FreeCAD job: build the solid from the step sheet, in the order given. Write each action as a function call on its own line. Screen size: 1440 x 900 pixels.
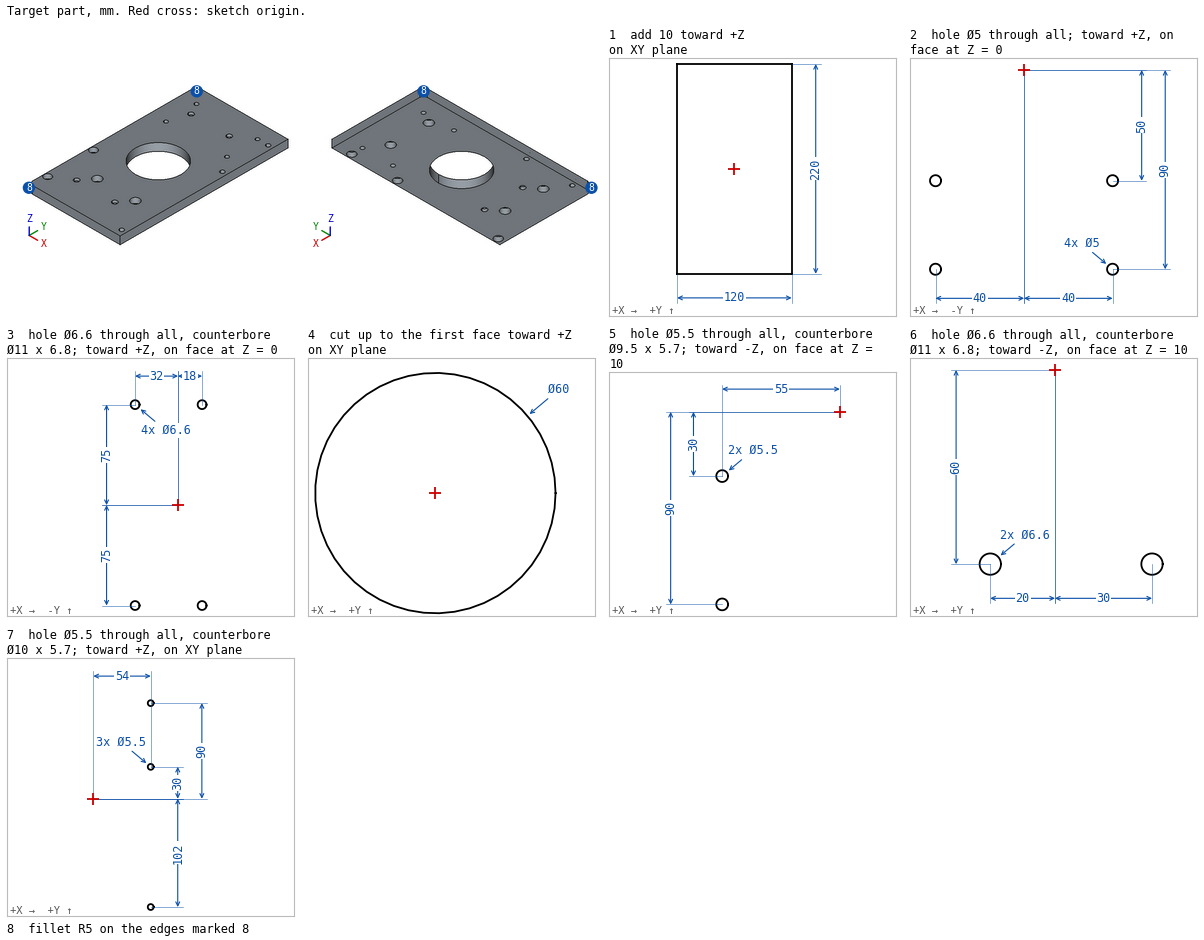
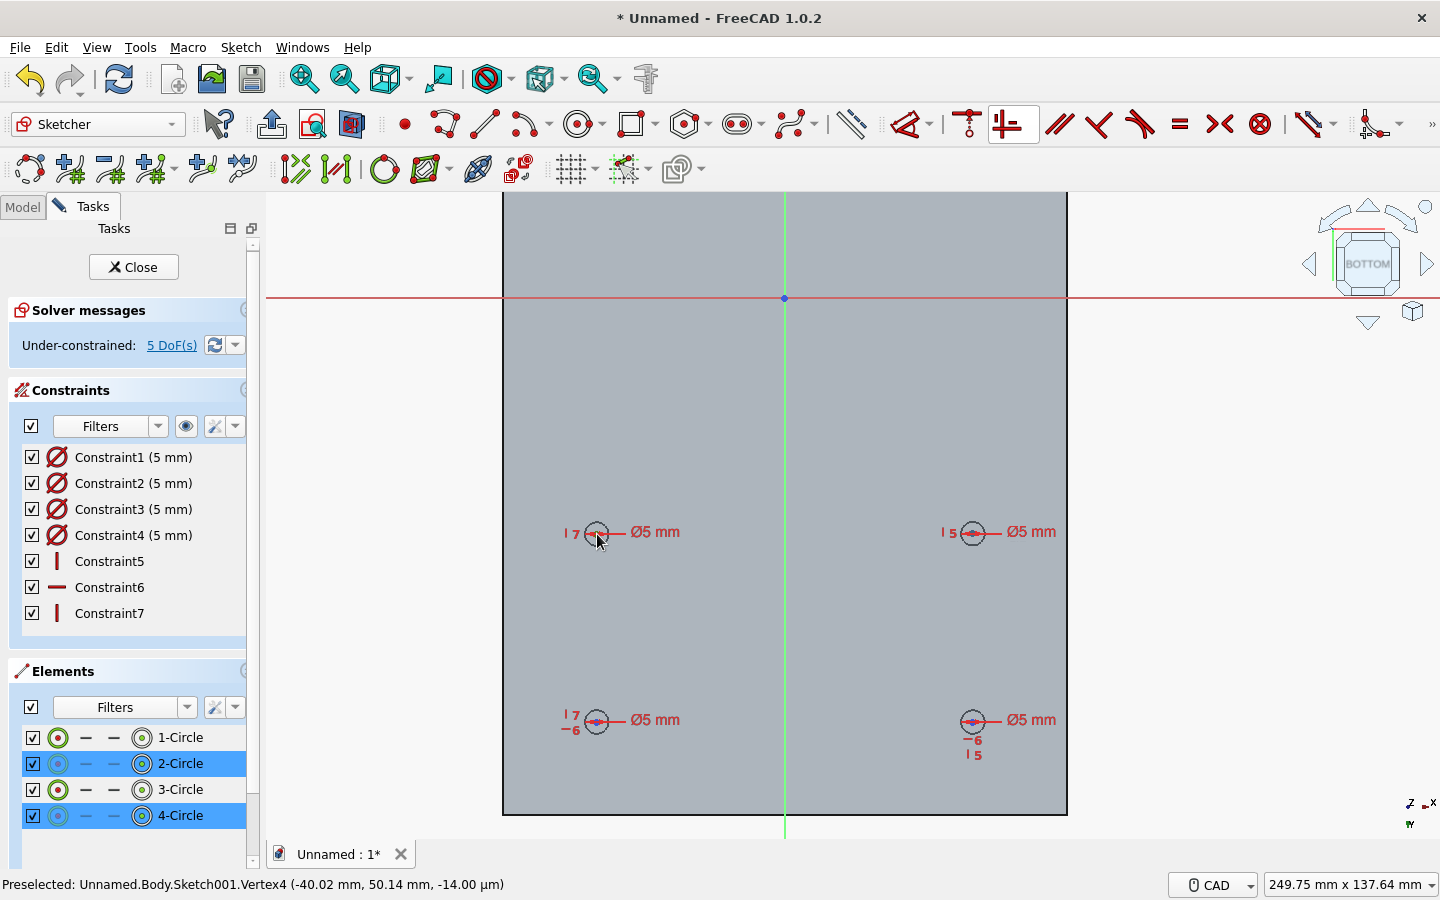
key(h)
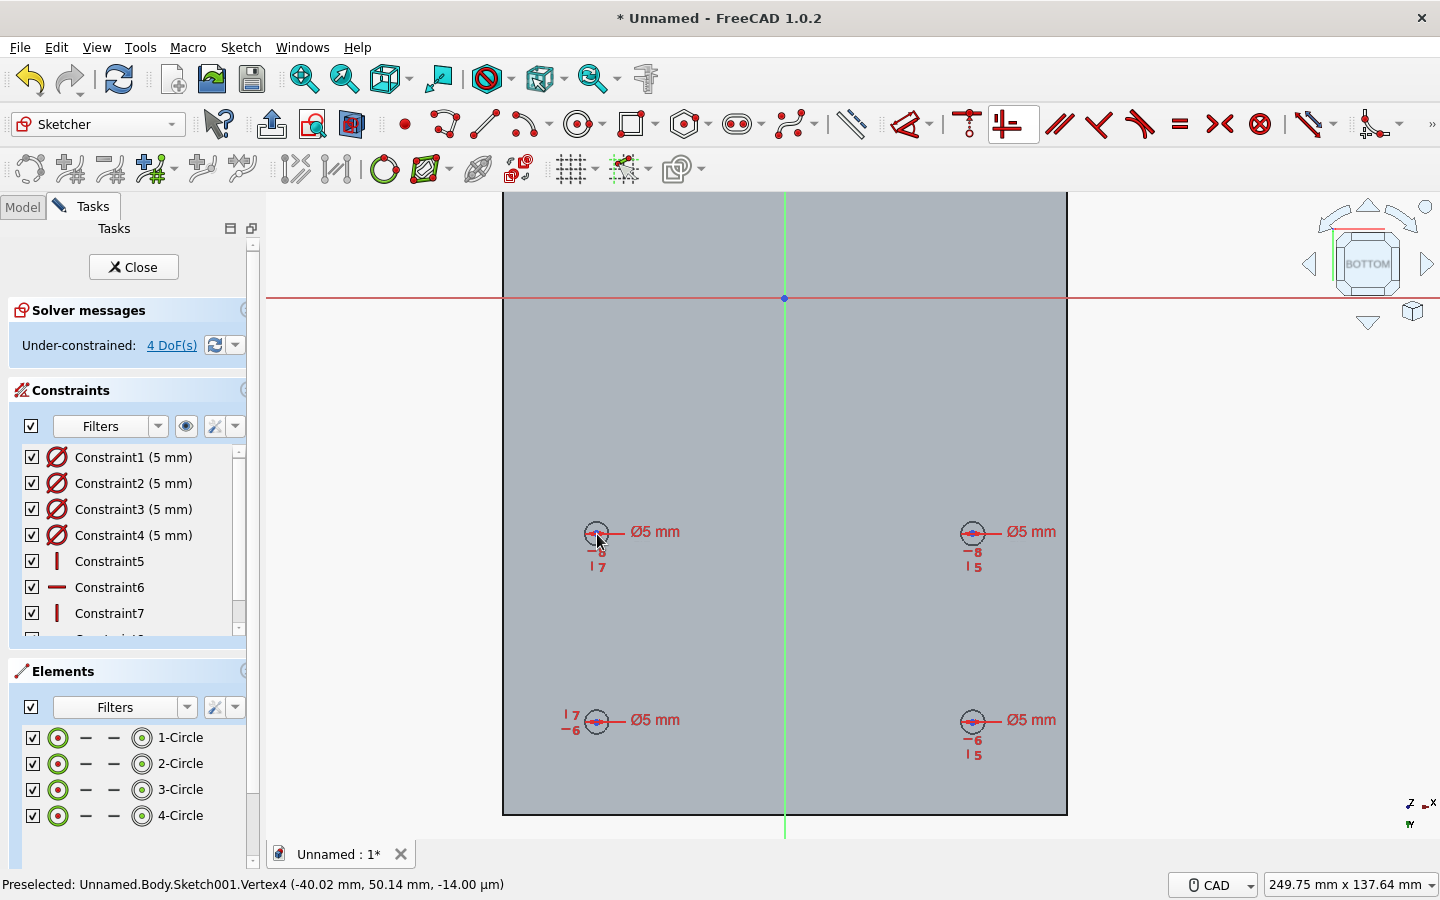
key(d)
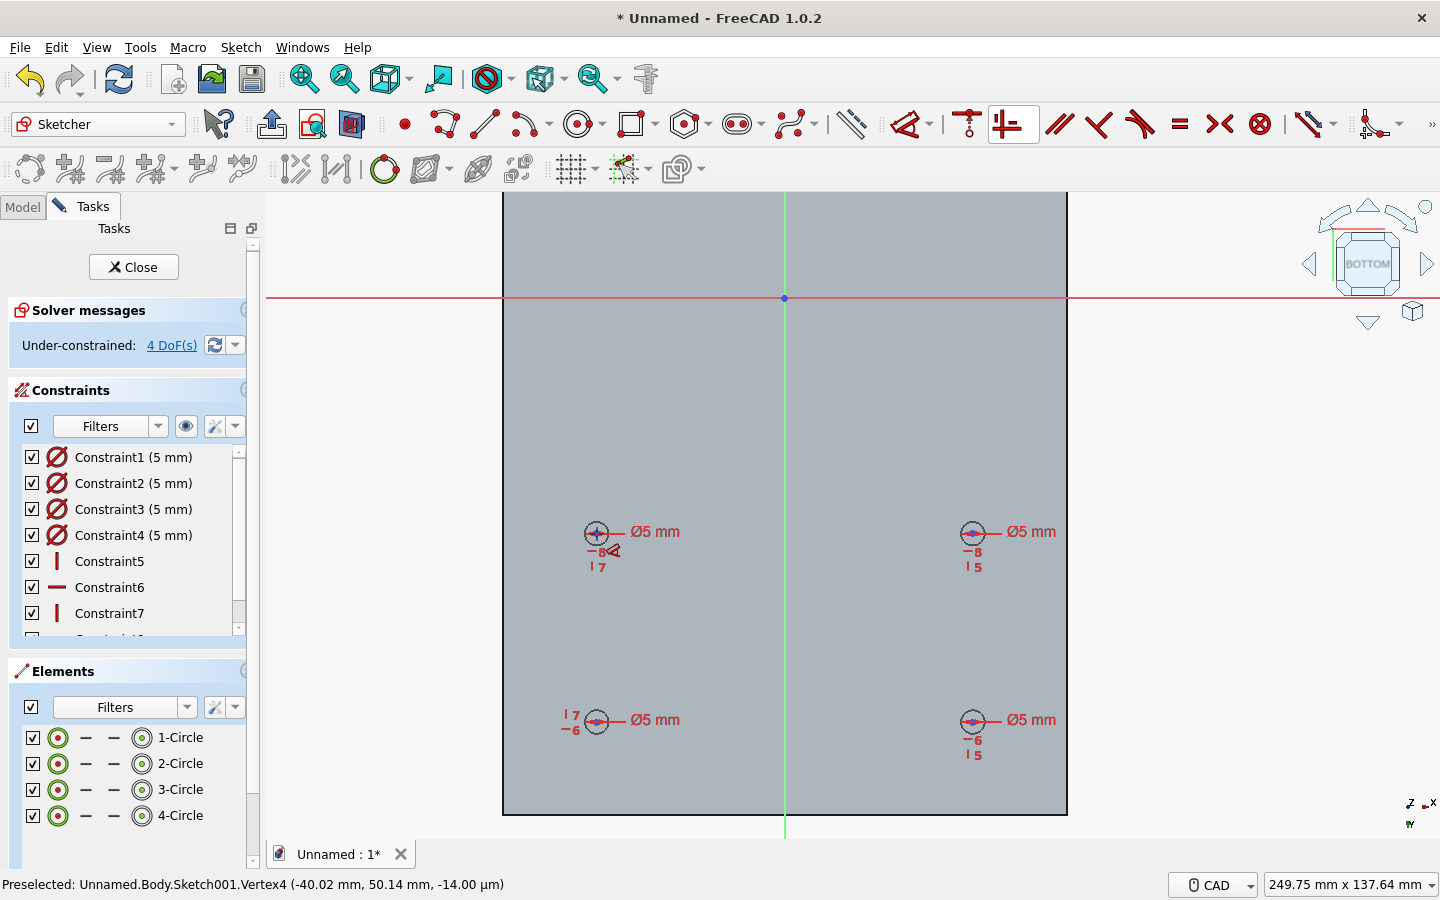
click(973, 722)
click(879, 264)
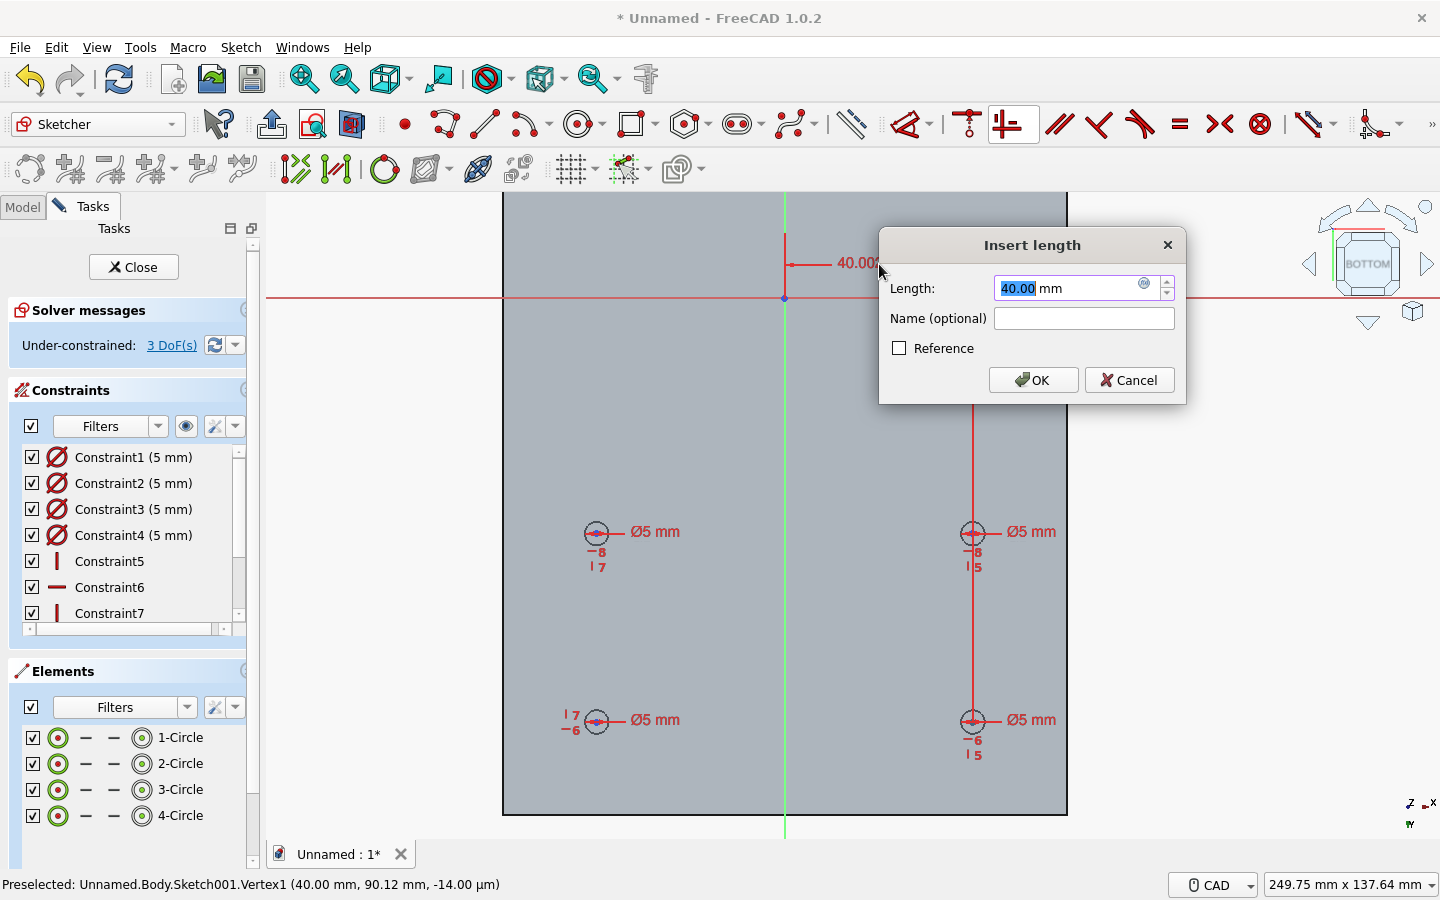
text(40)
key(Return)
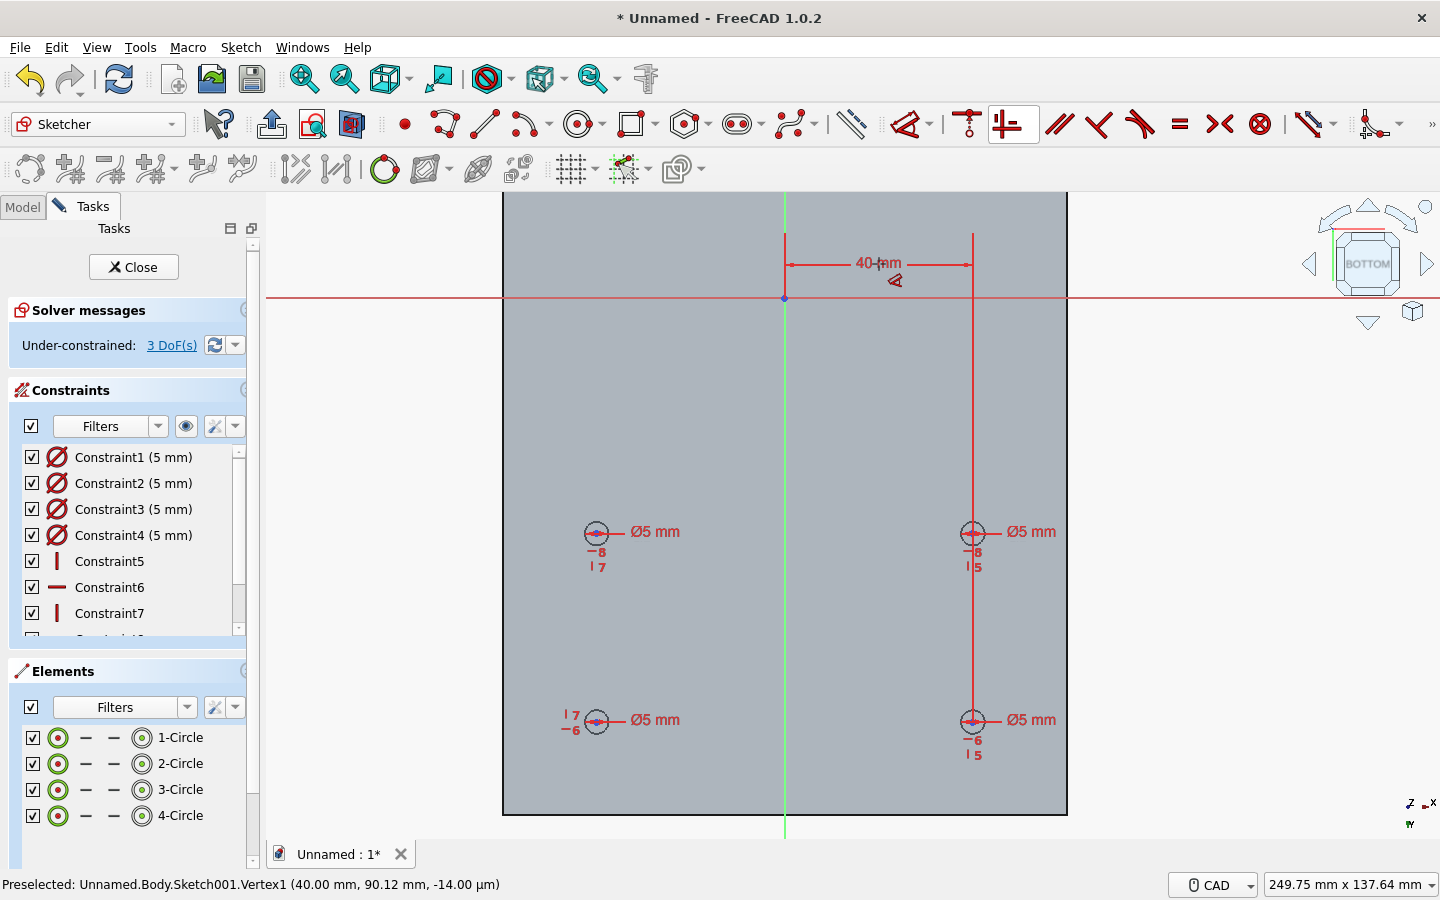
click(973, 722)
click(1007, 510)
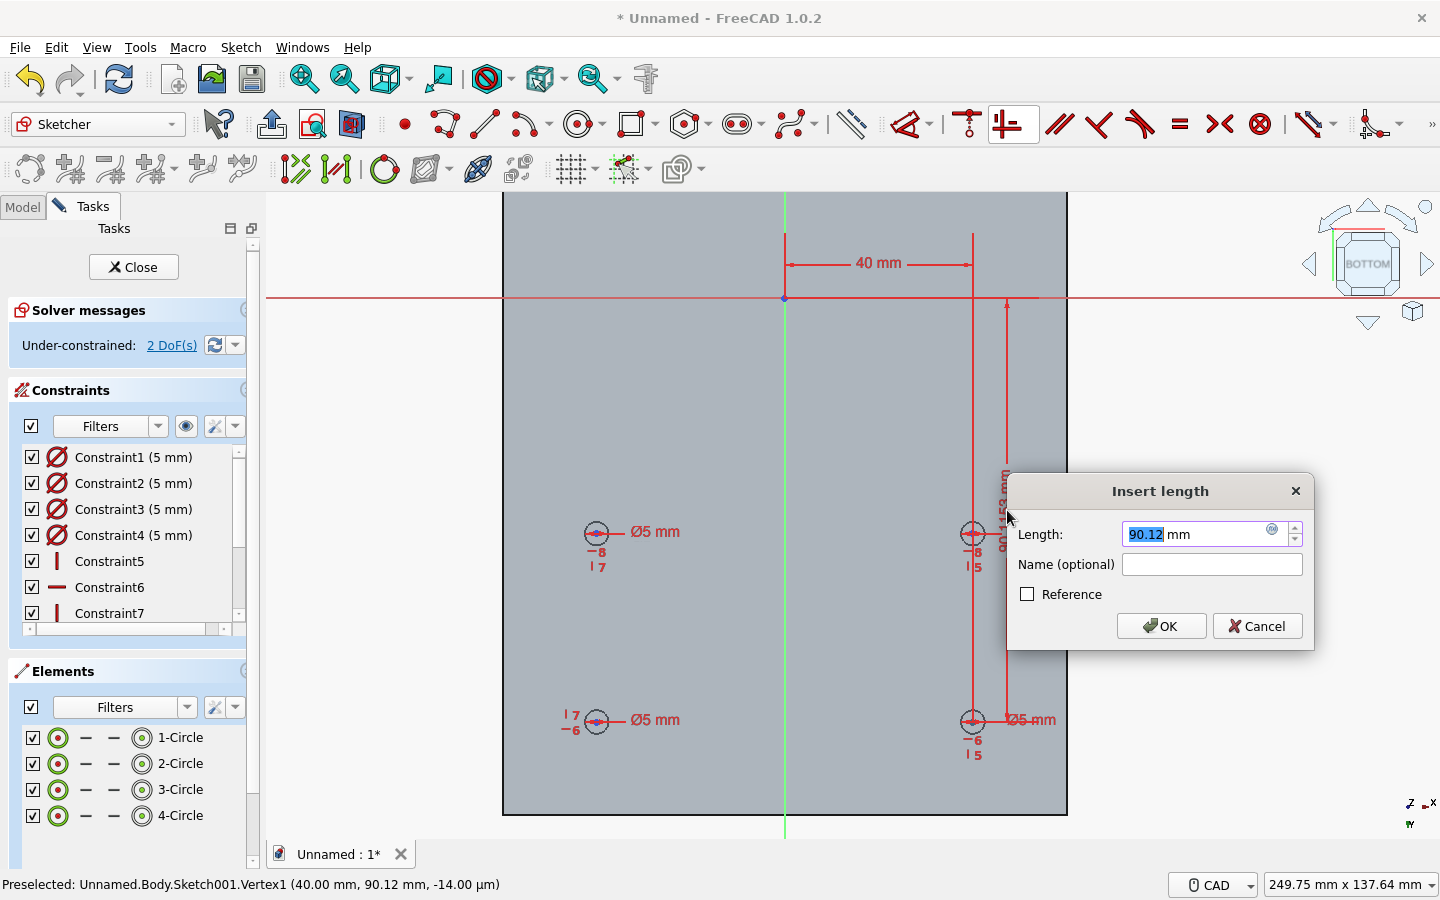
text(90)
key(Return)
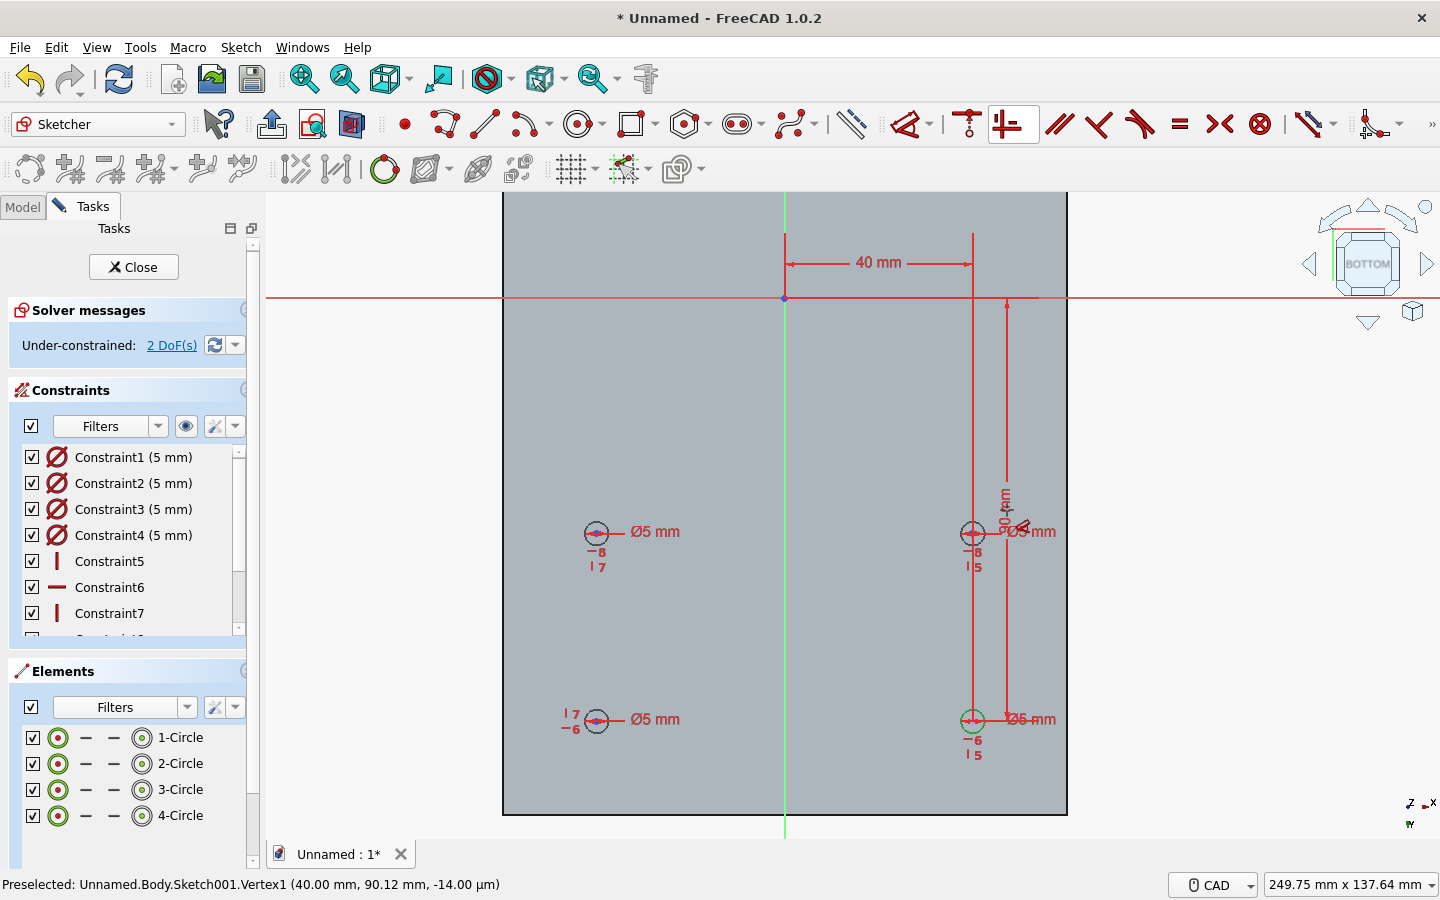
click(973, 534)
click(1007, 416)